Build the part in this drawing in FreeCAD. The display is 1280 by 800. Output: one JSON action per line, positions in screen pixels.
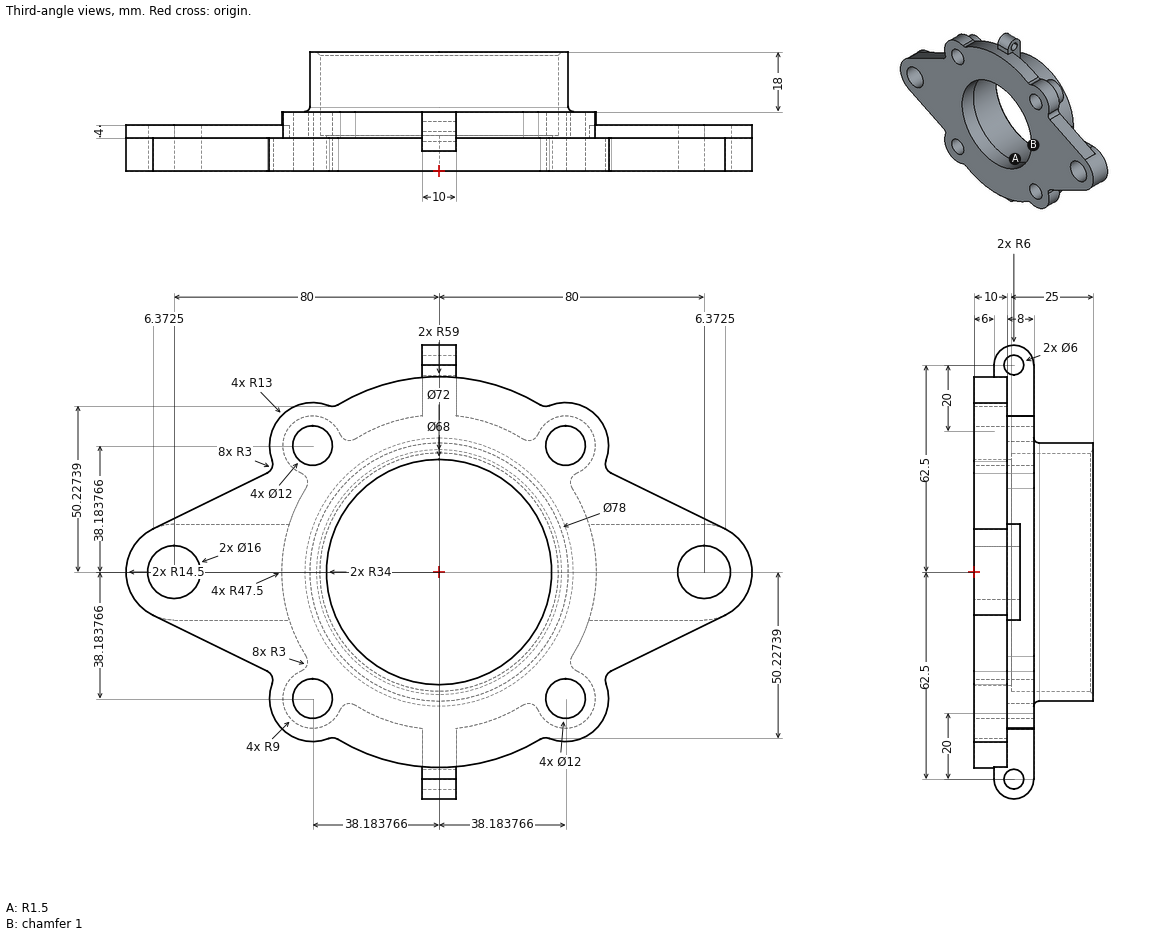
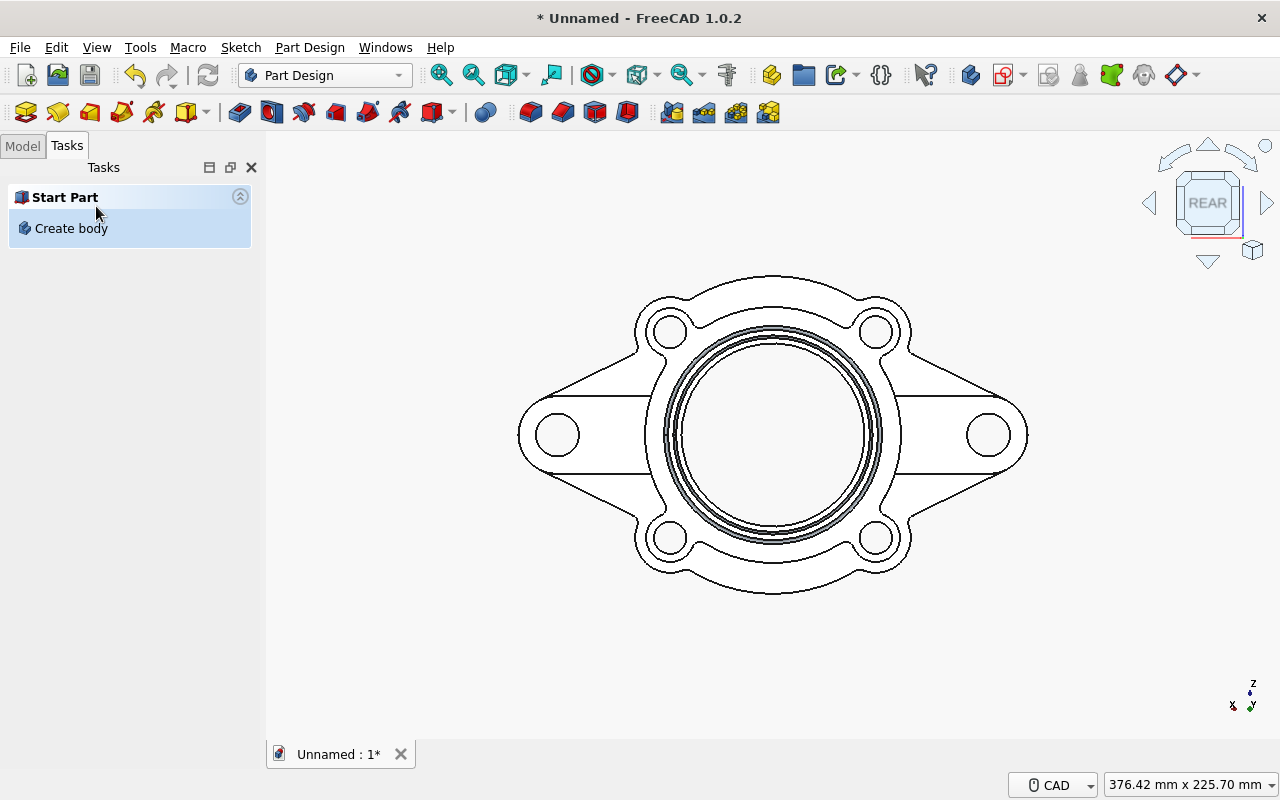
{"action": "left_click", "coordinate": [1004, 76]}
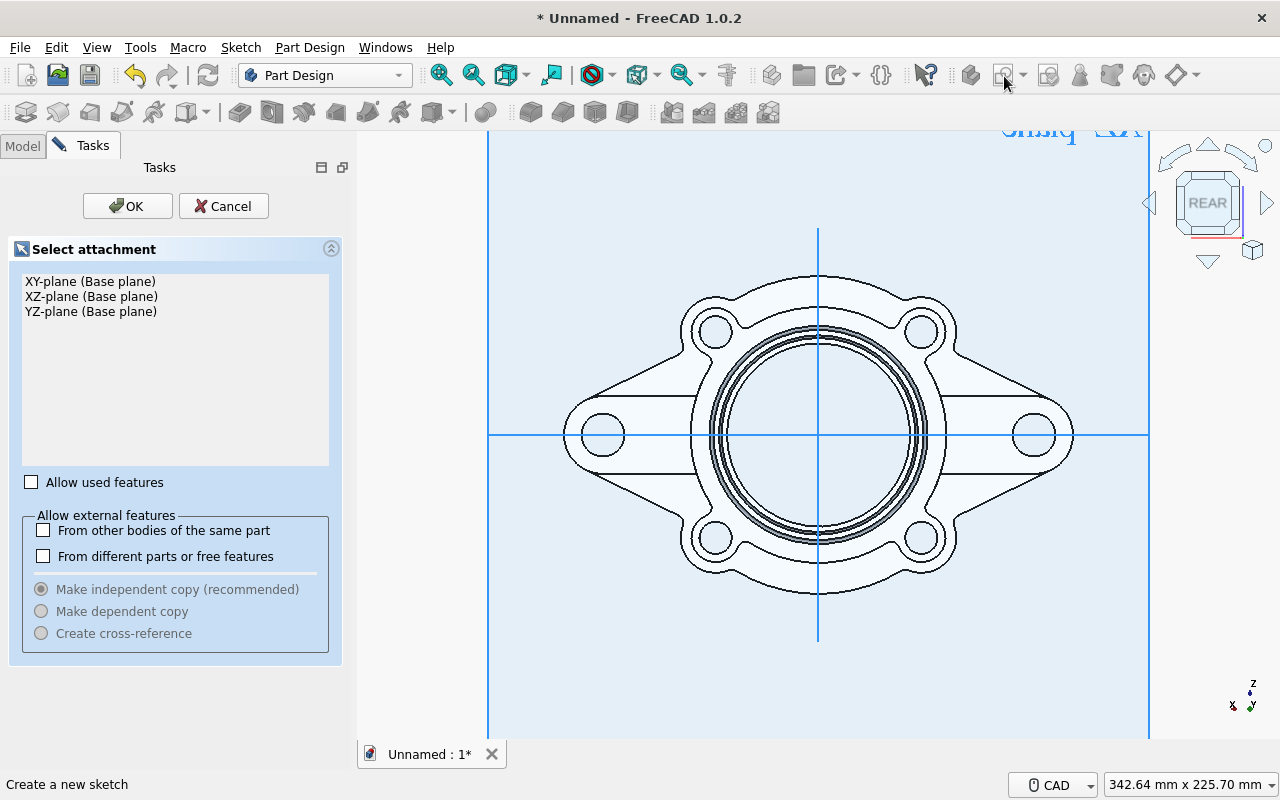
{"action": "left_click", "coordinate": [82, 312]}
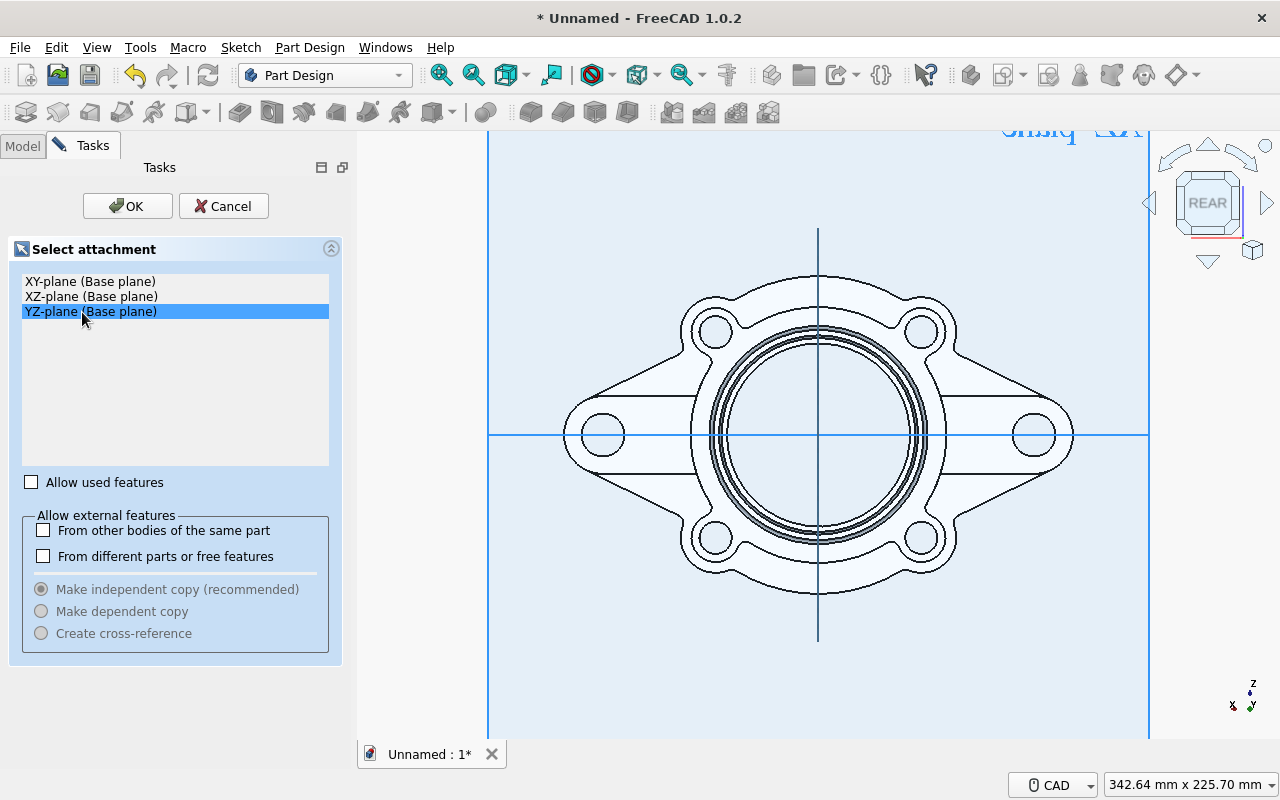
{"action": "left_click", "coordinate": [128, 206]}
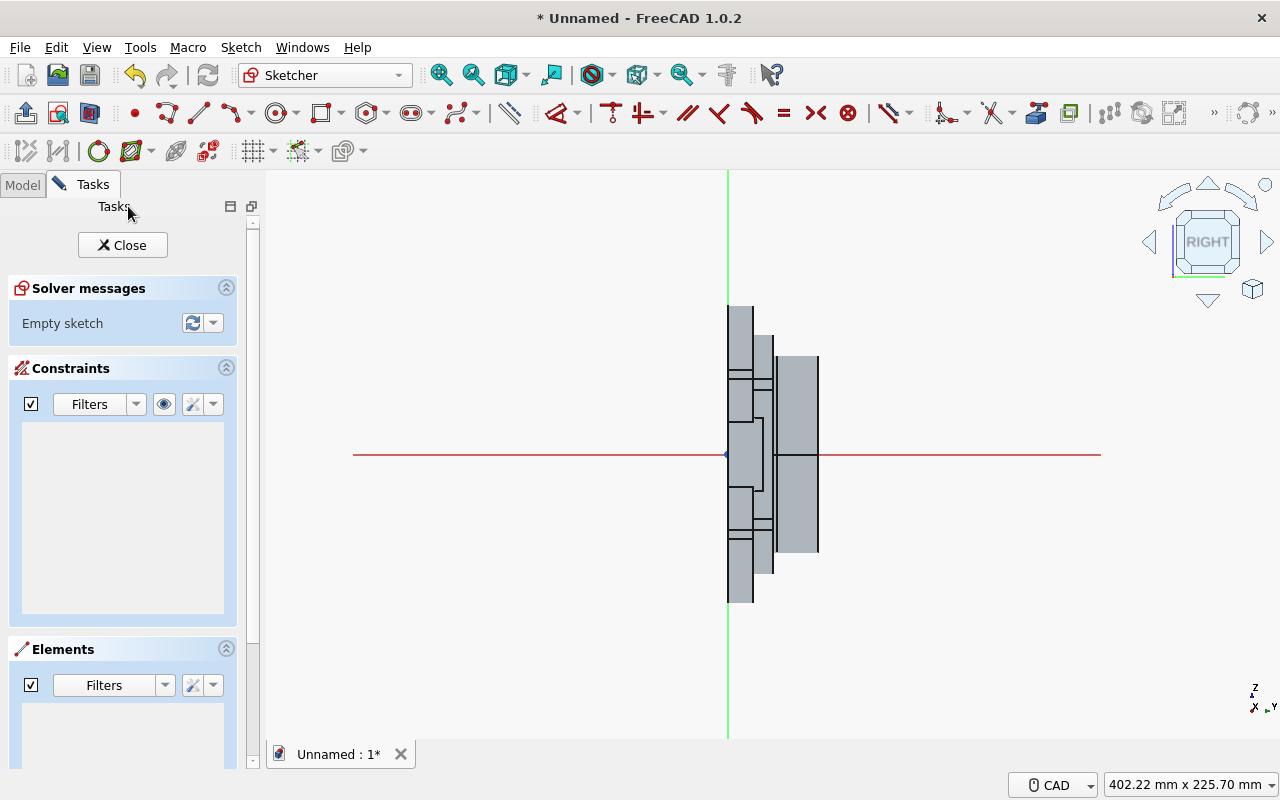
{"action": "left_click", "coordinate": [90, 114]}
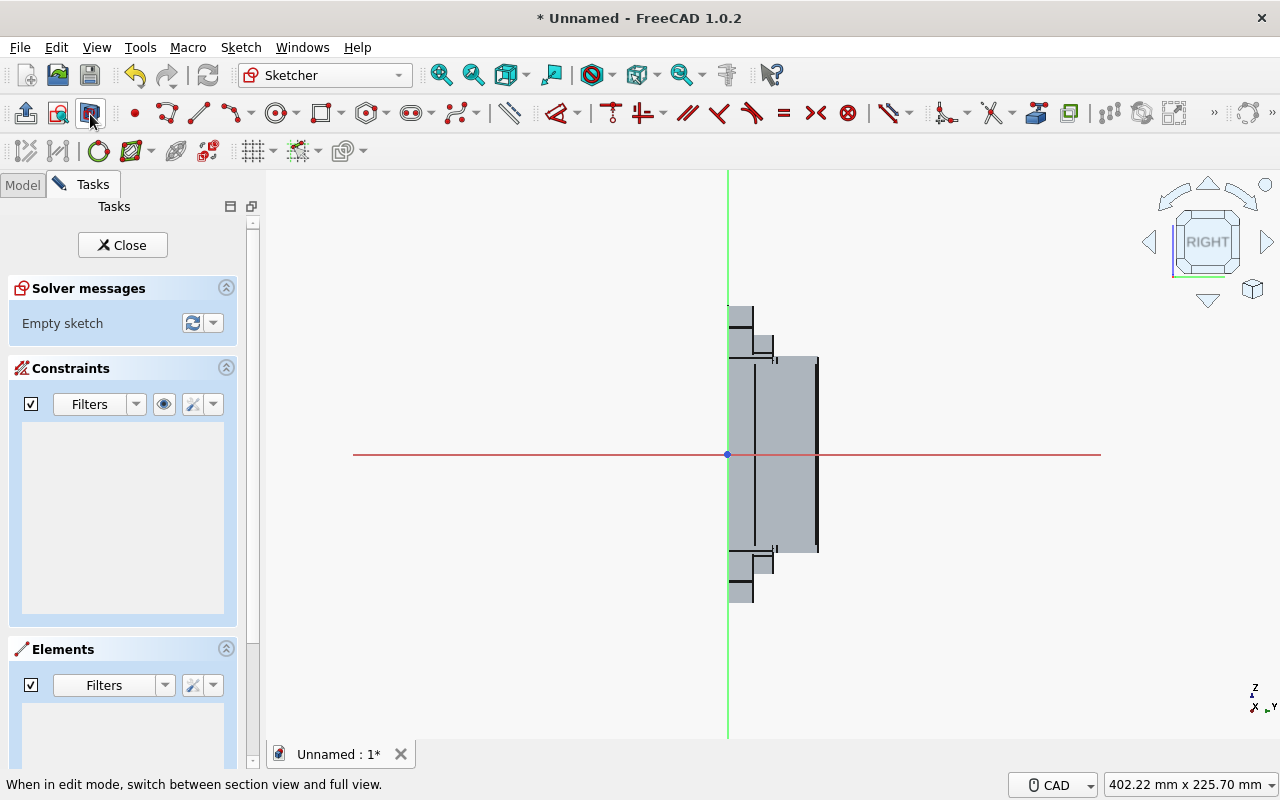
{"action": "left_click", "coordinate": [168, 114]}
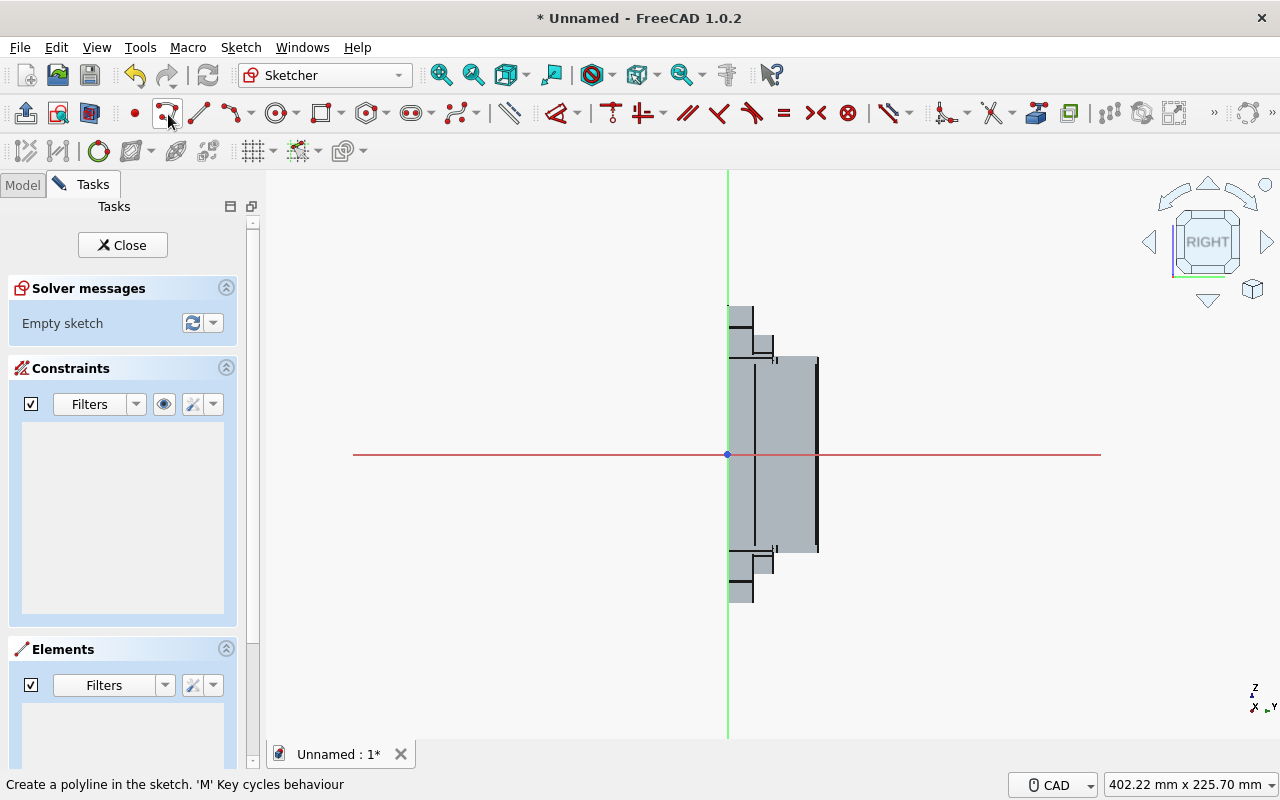
{"action": "left_click", "coordinate": [743, 297]}
{"action": "left_click", "coordinate": [743, 347]}
{"action": "left_click", "coordinate": [773, 347]}
{"action": "left_click", "coordinate": [773, 297]}
{"action": "right_click", "coordinate": [773, 297]}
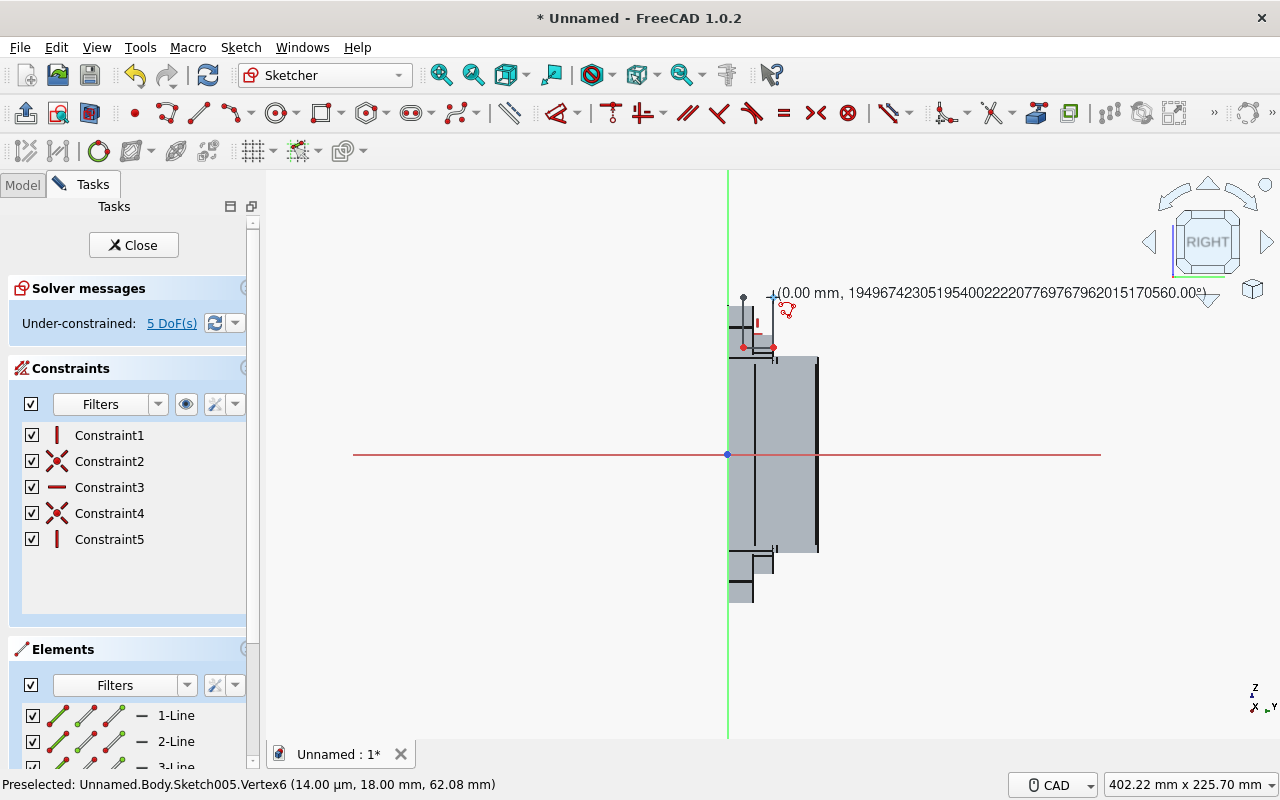
{"action": "left_click", "coordinate": [232, 114]}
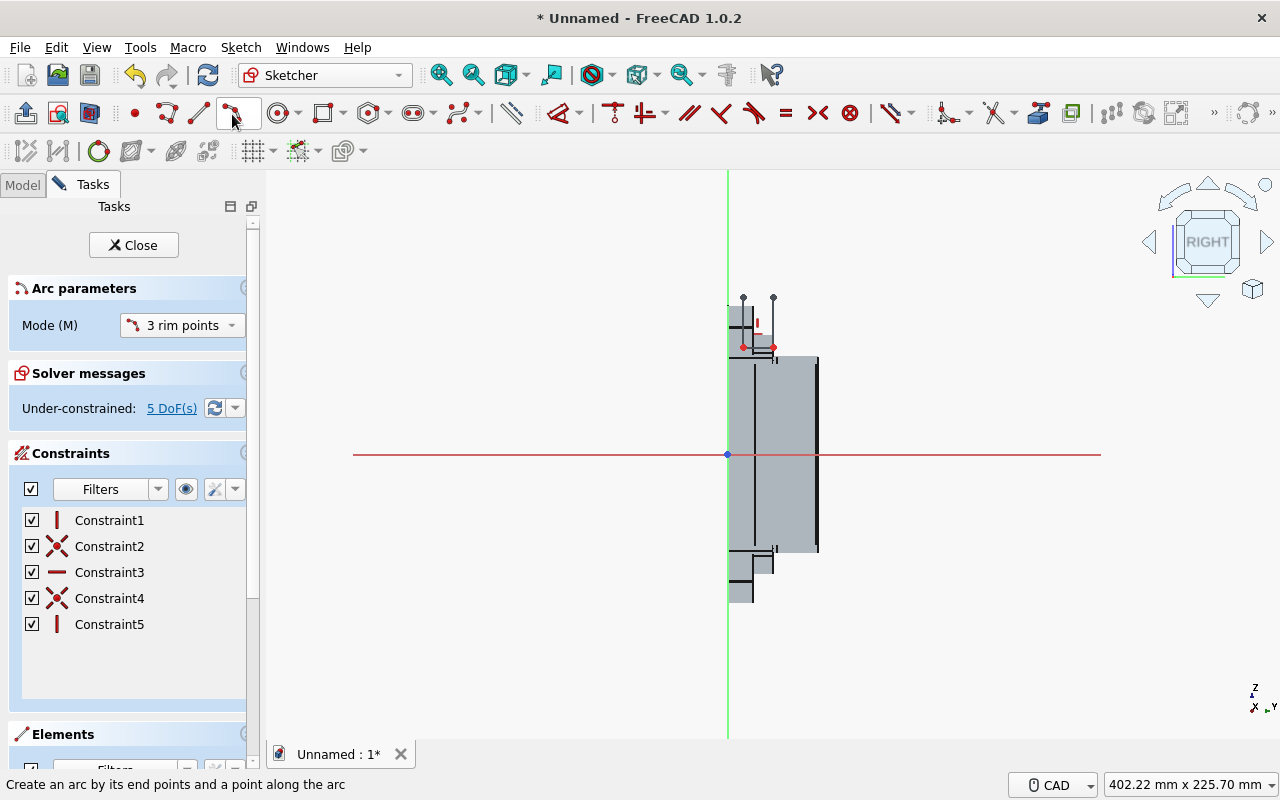
{"action": "left_click", "coordinate": [773, 298]}
{"action": "left_click", "coordinate": [743, 298]}
{"action": "left_click", "coordinate": [758, 282]}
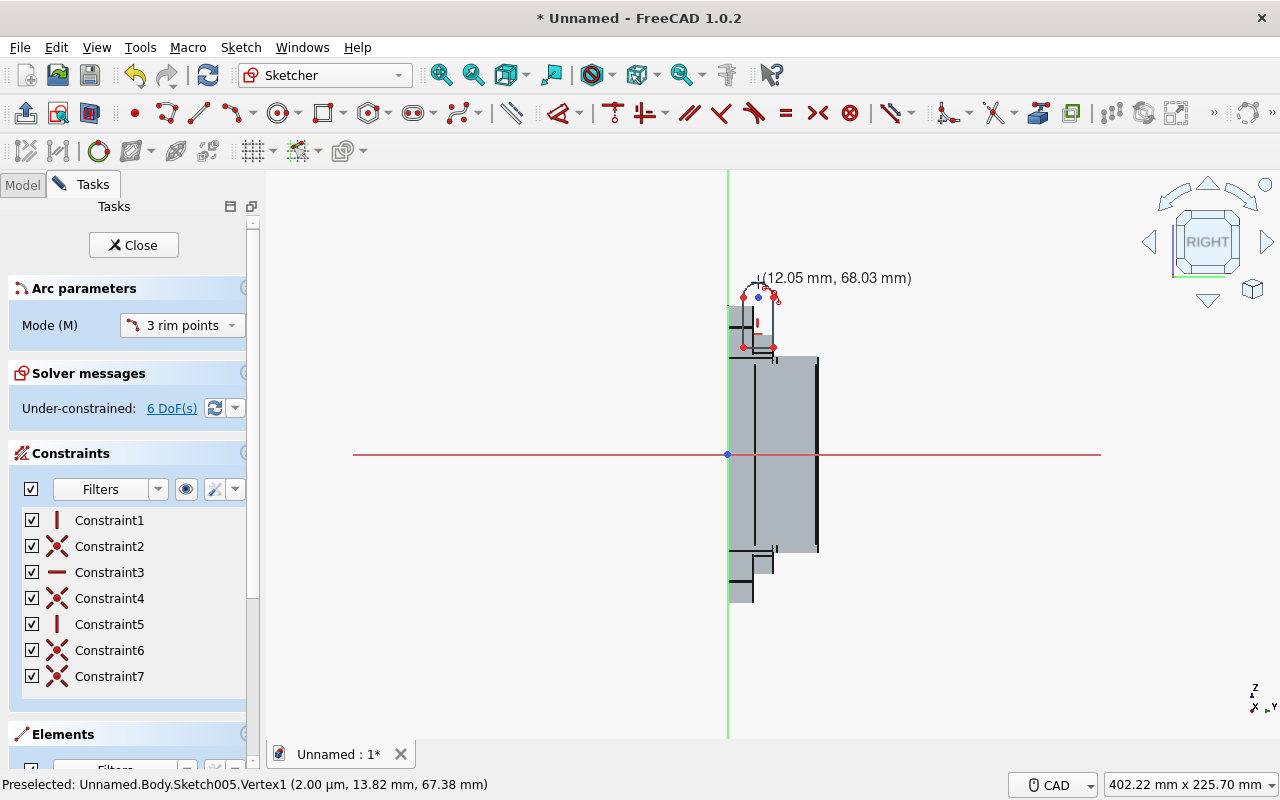
{"action": "left_click", "coordinate": [168, 114]}